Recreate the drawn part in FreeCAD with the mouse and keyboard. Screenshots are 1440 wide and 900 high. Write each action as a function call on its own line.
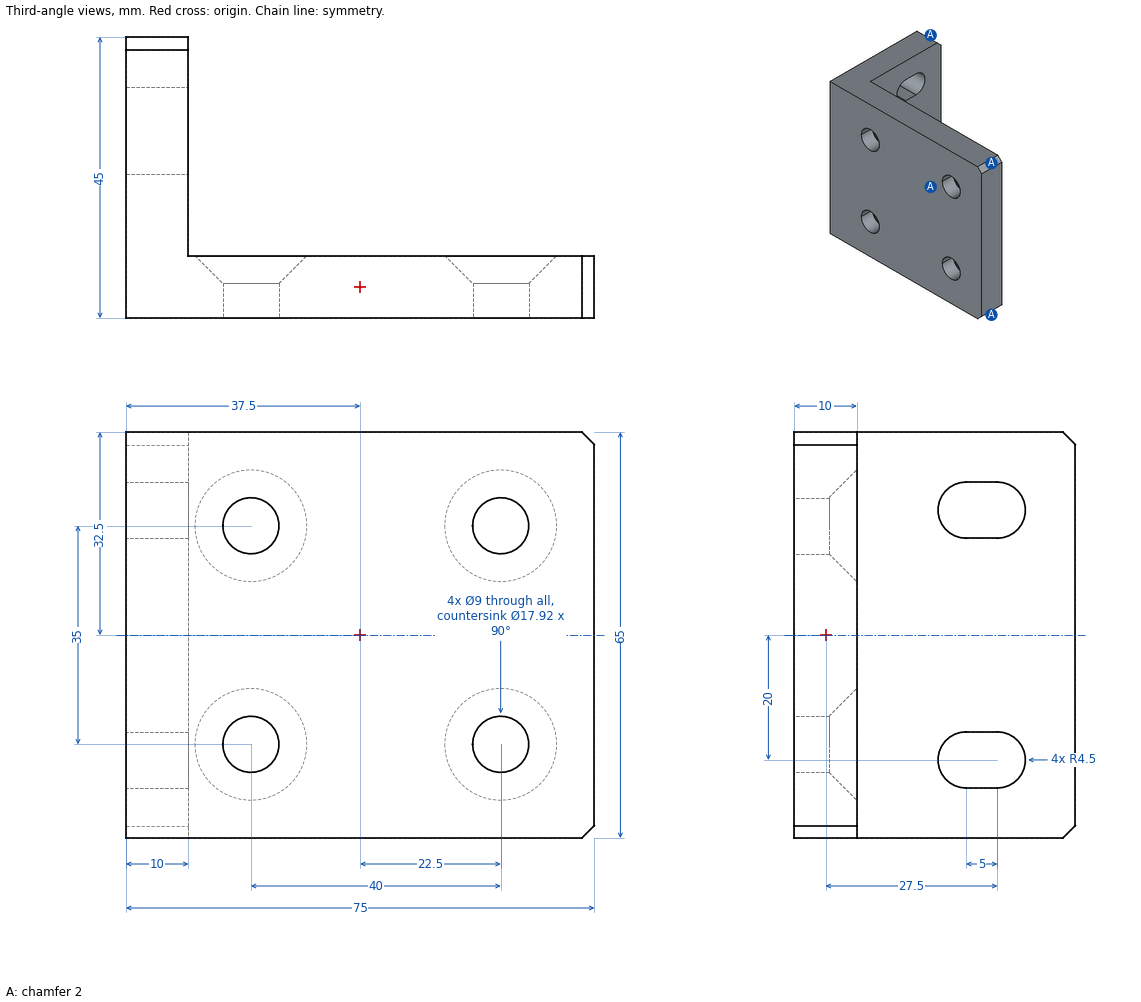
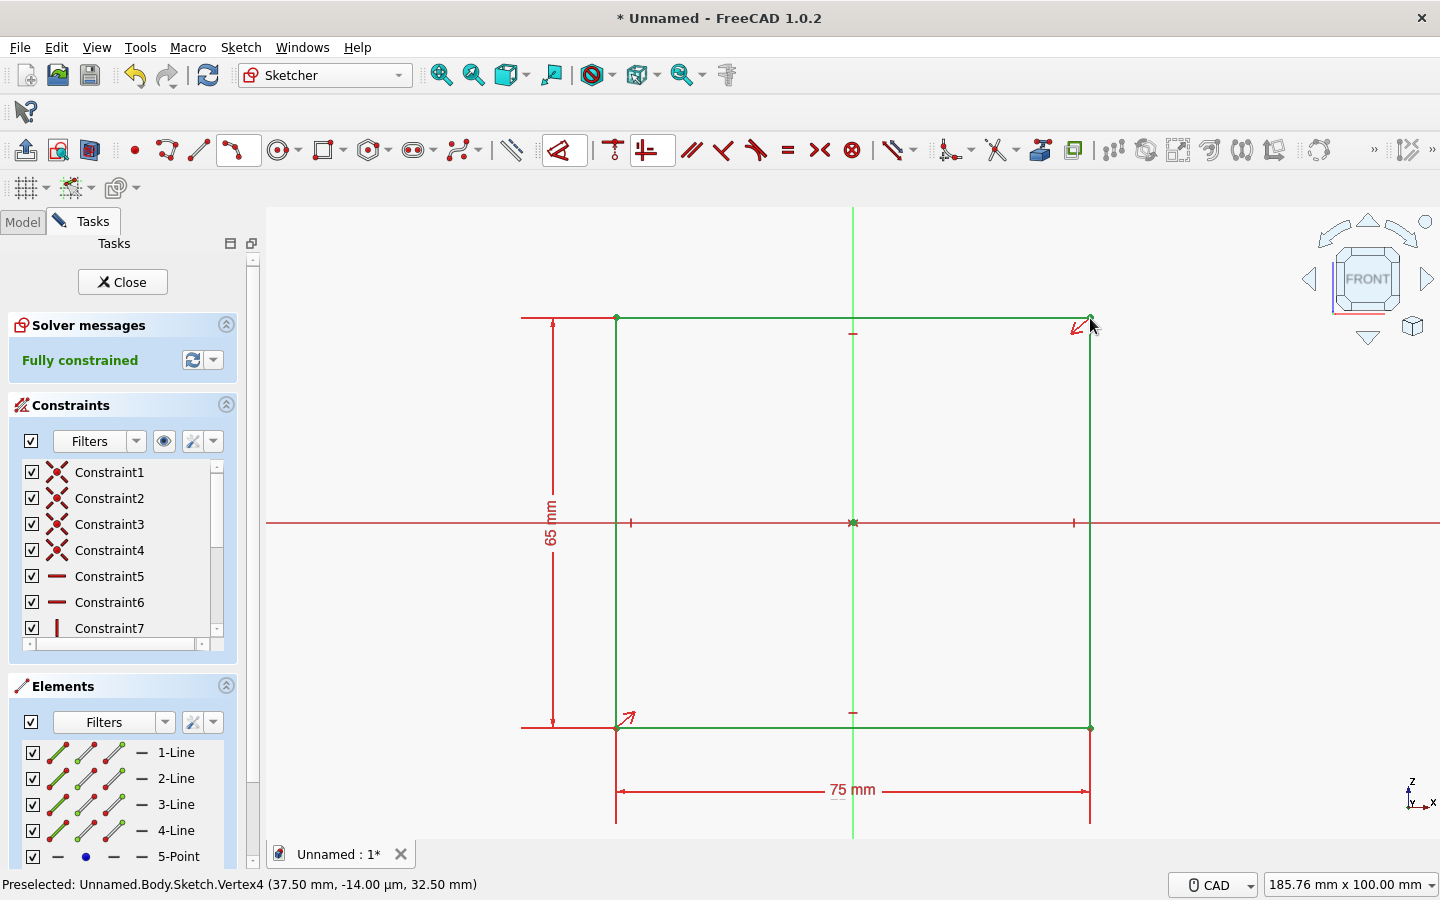
click(123, 282)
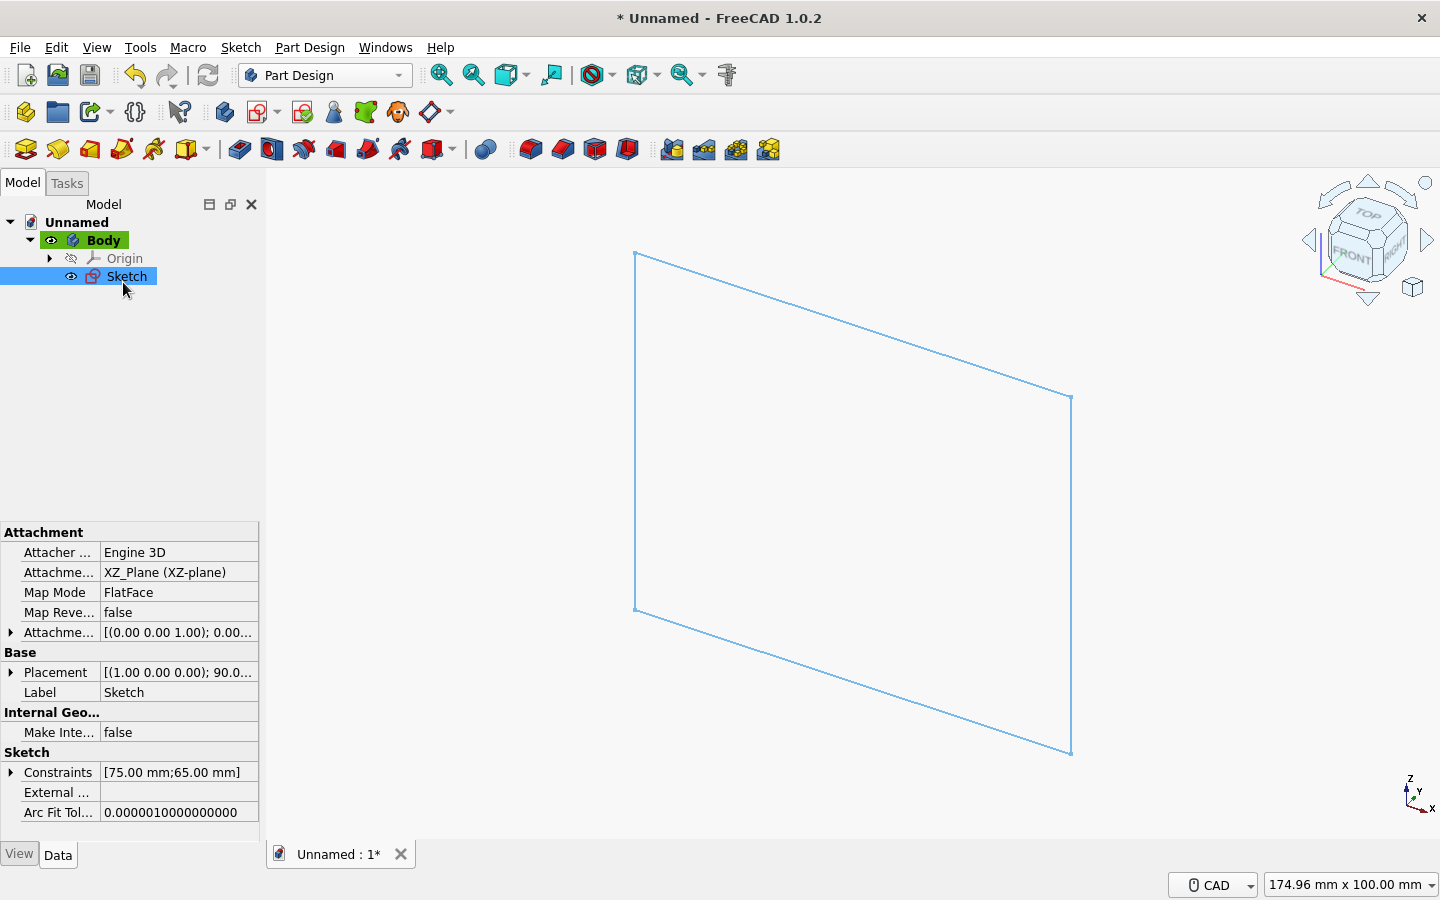
click(26, 150)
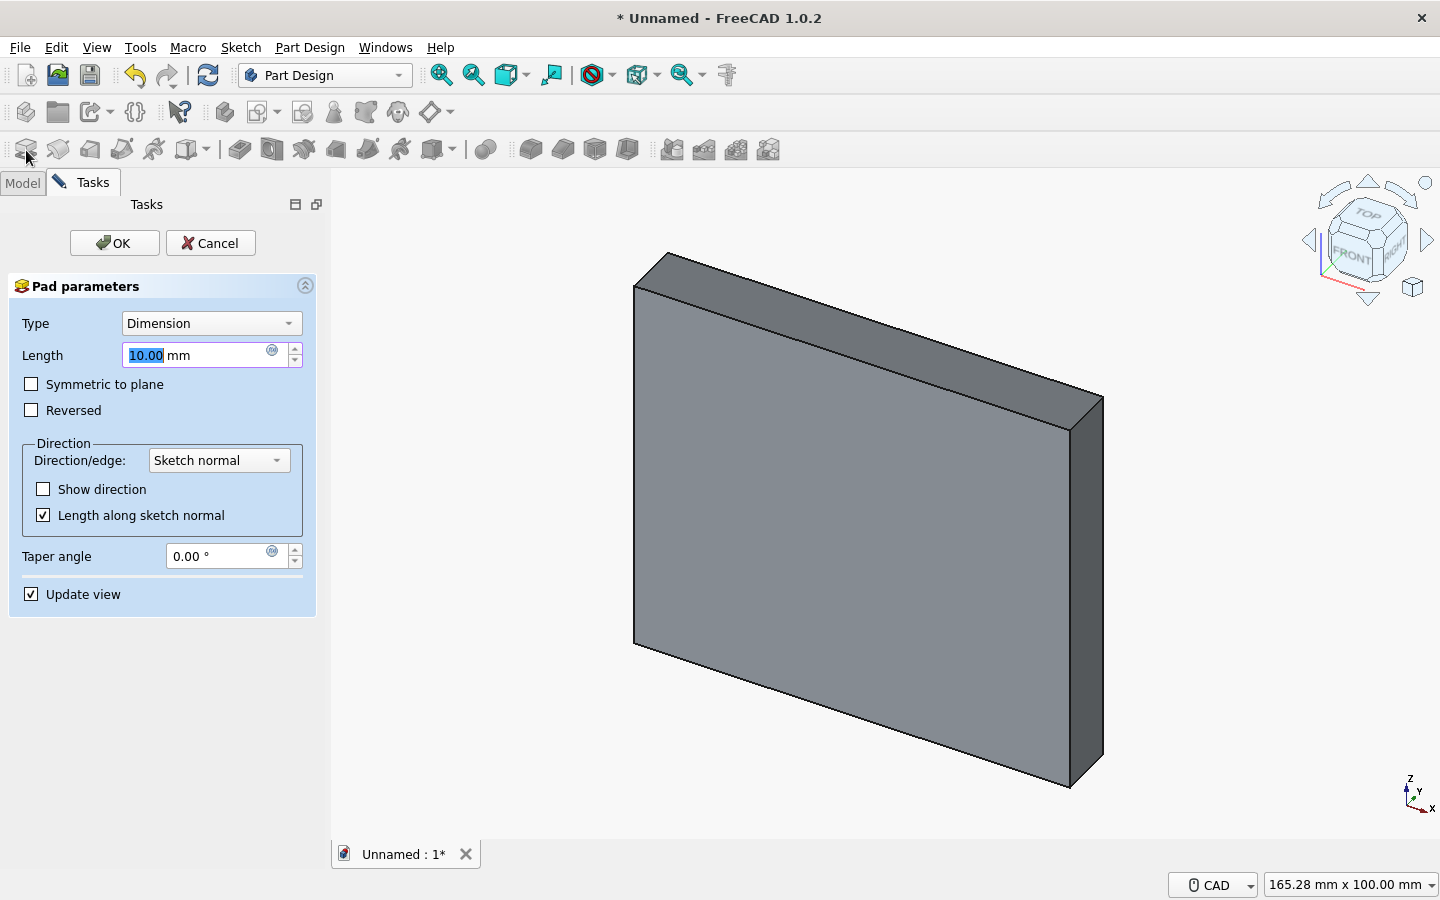
text(10)
key(Tab)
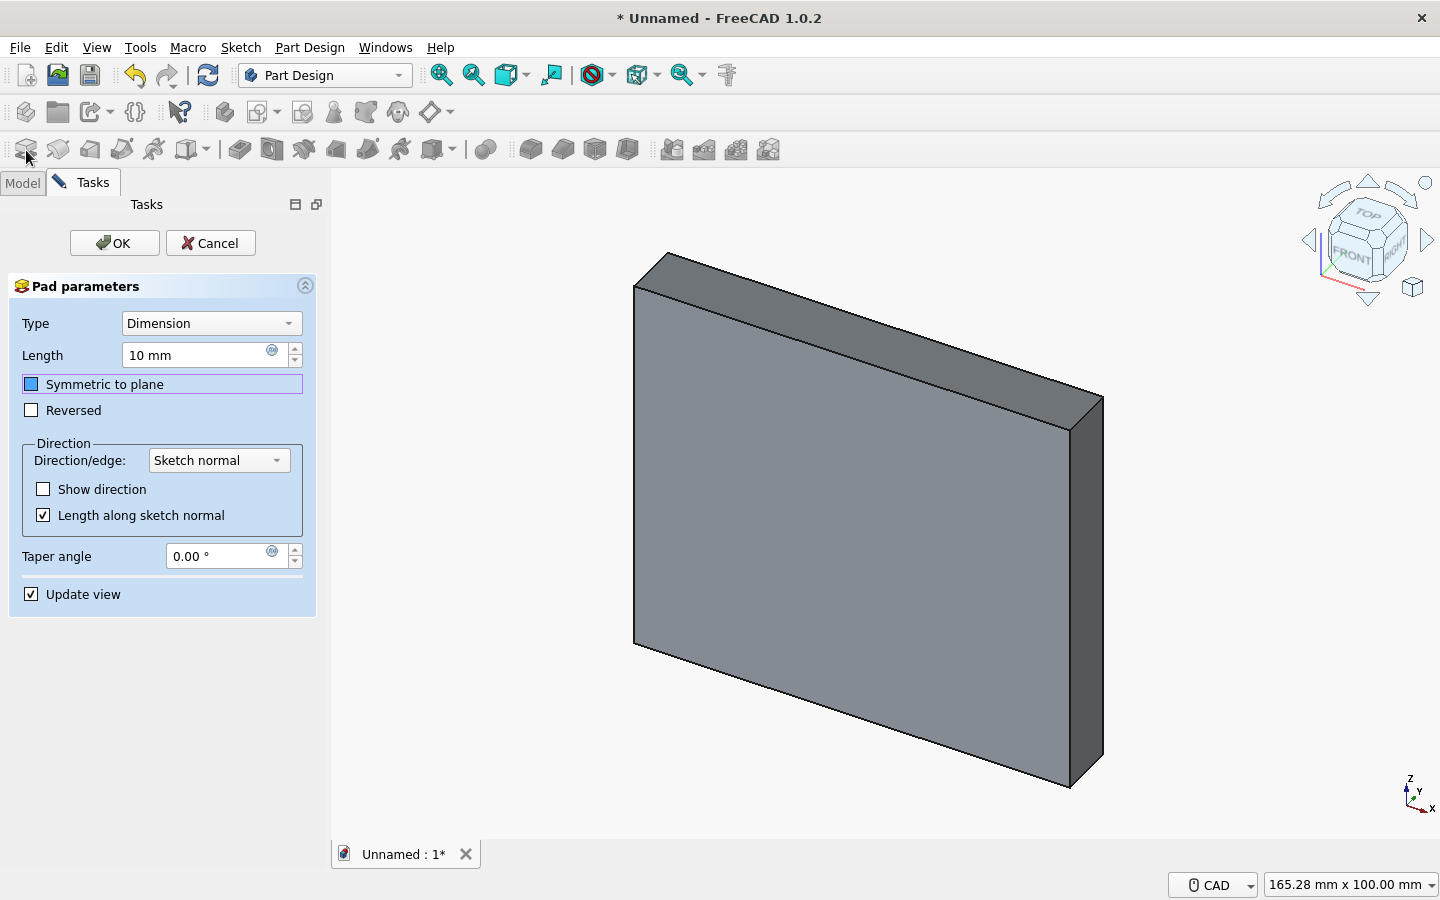
click(30, 384)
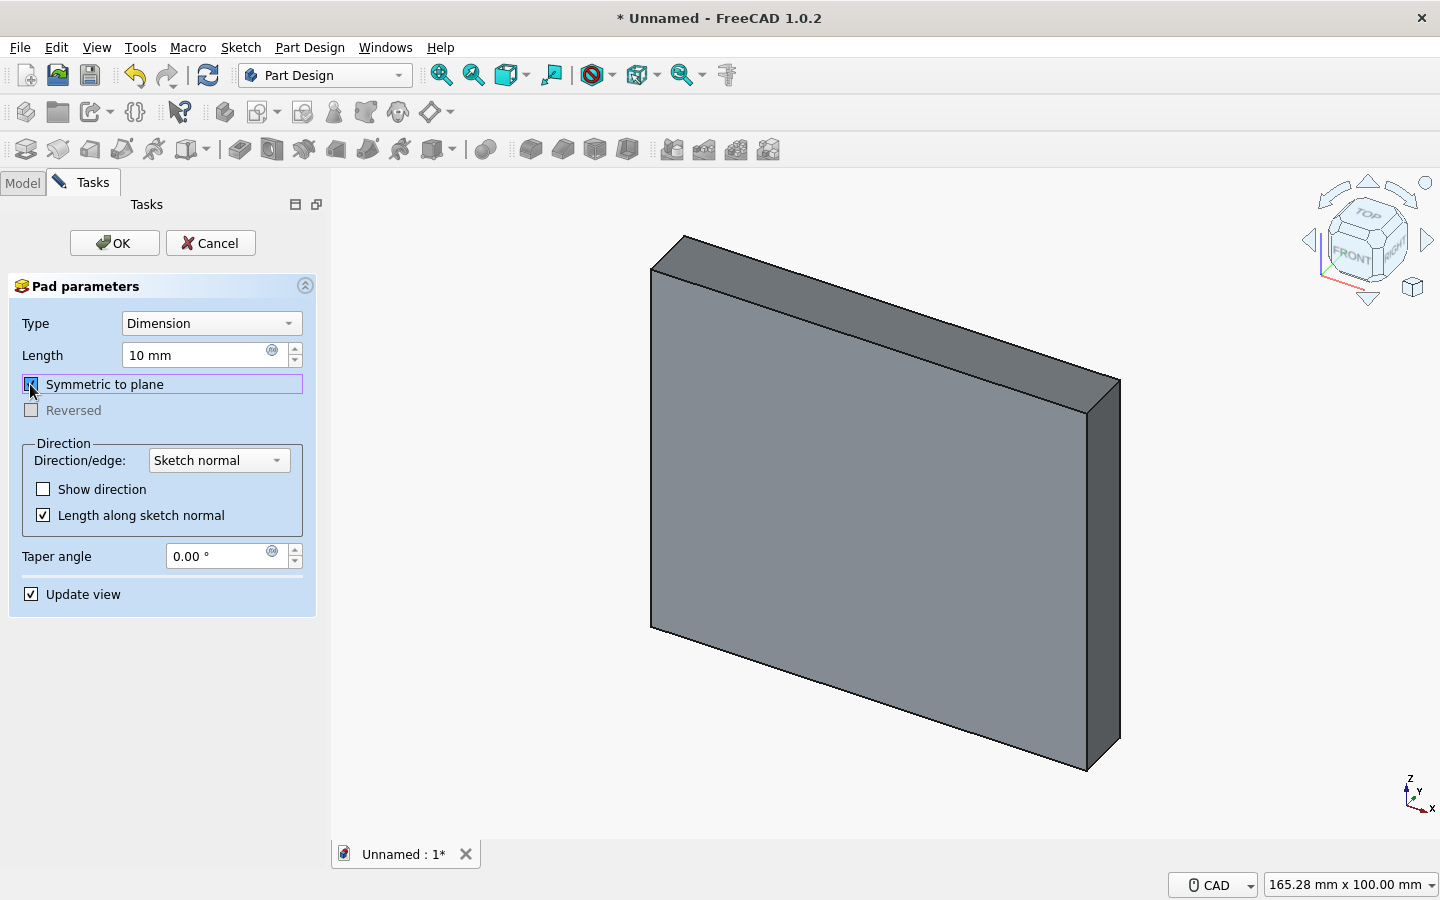
click(115, 243)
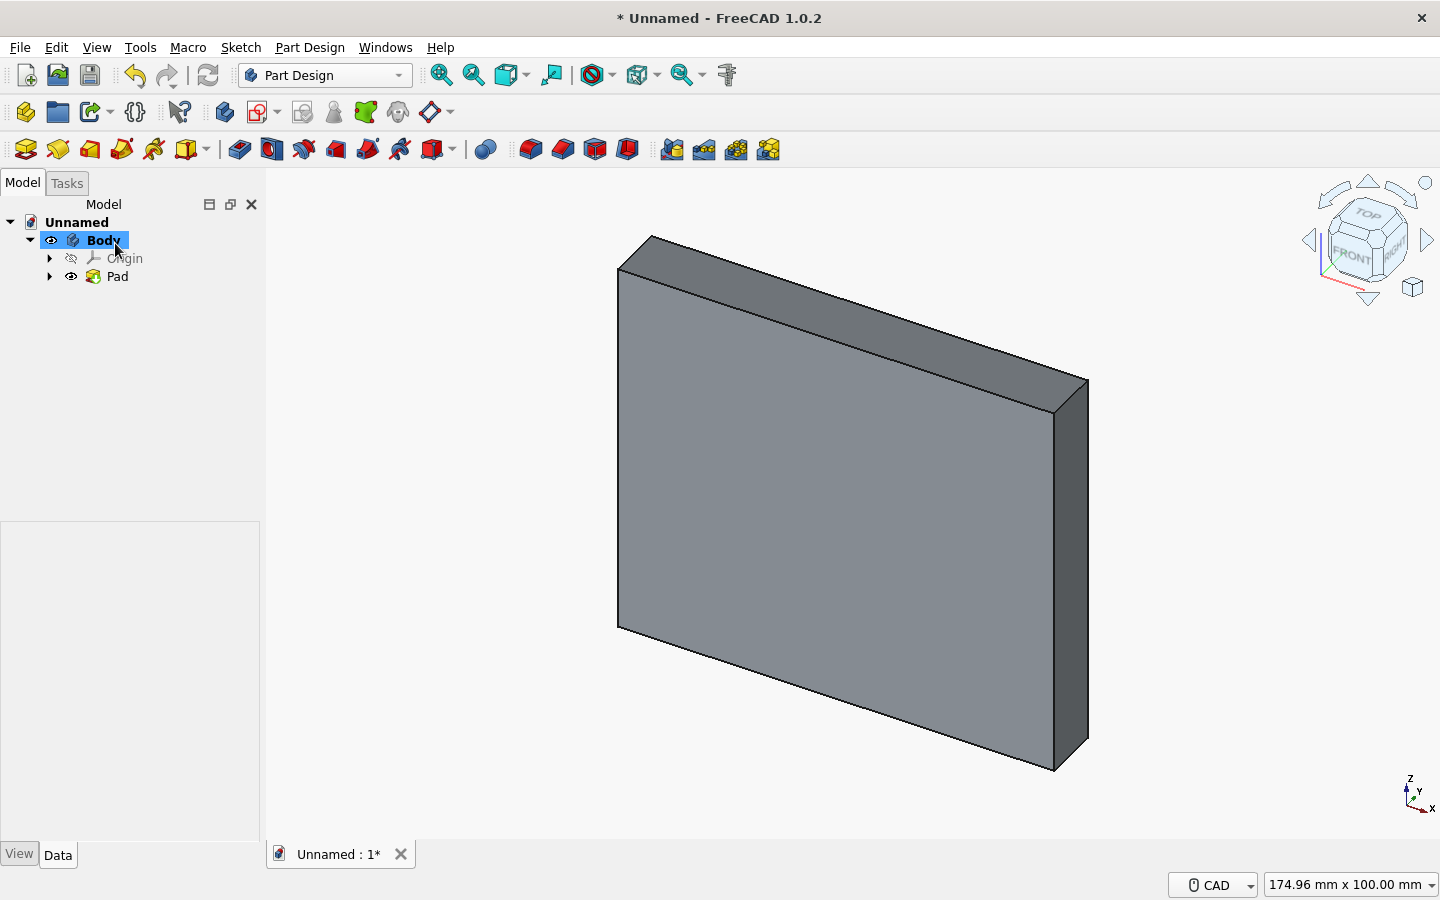
click(836, 519)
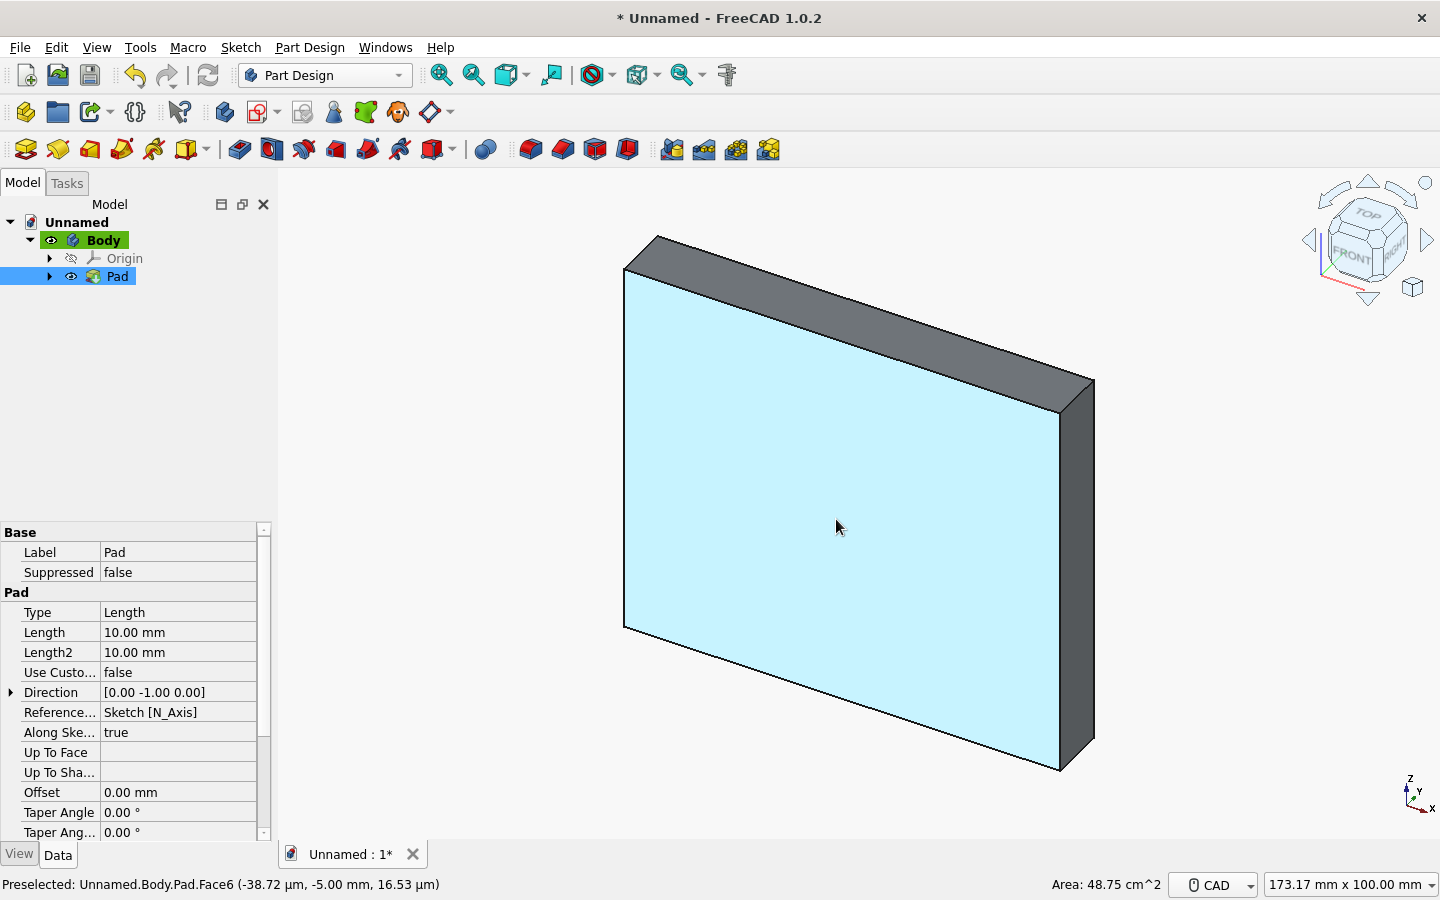
click(258, 112)